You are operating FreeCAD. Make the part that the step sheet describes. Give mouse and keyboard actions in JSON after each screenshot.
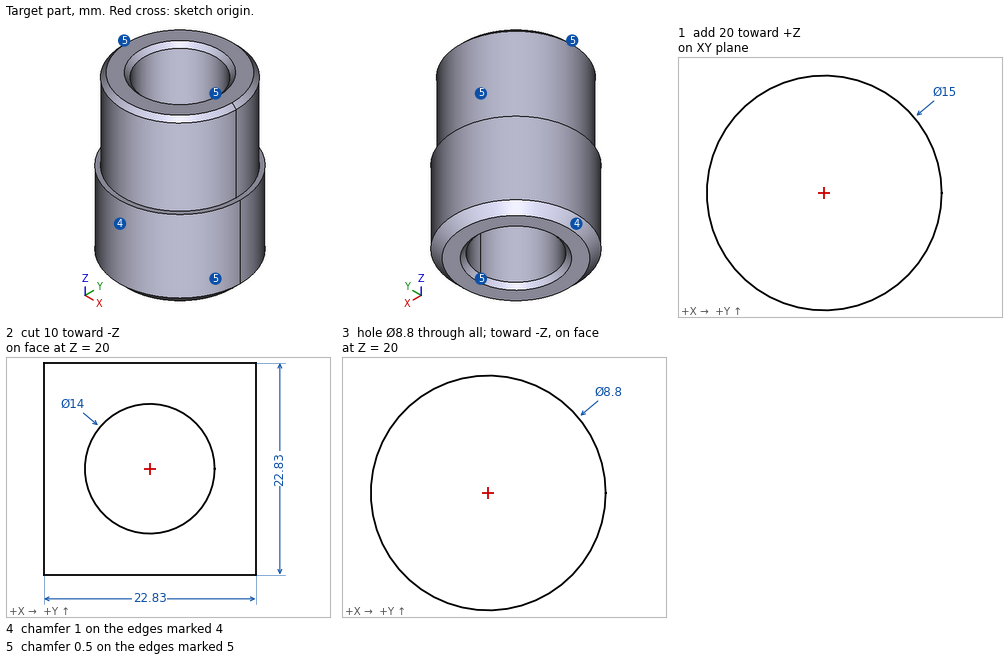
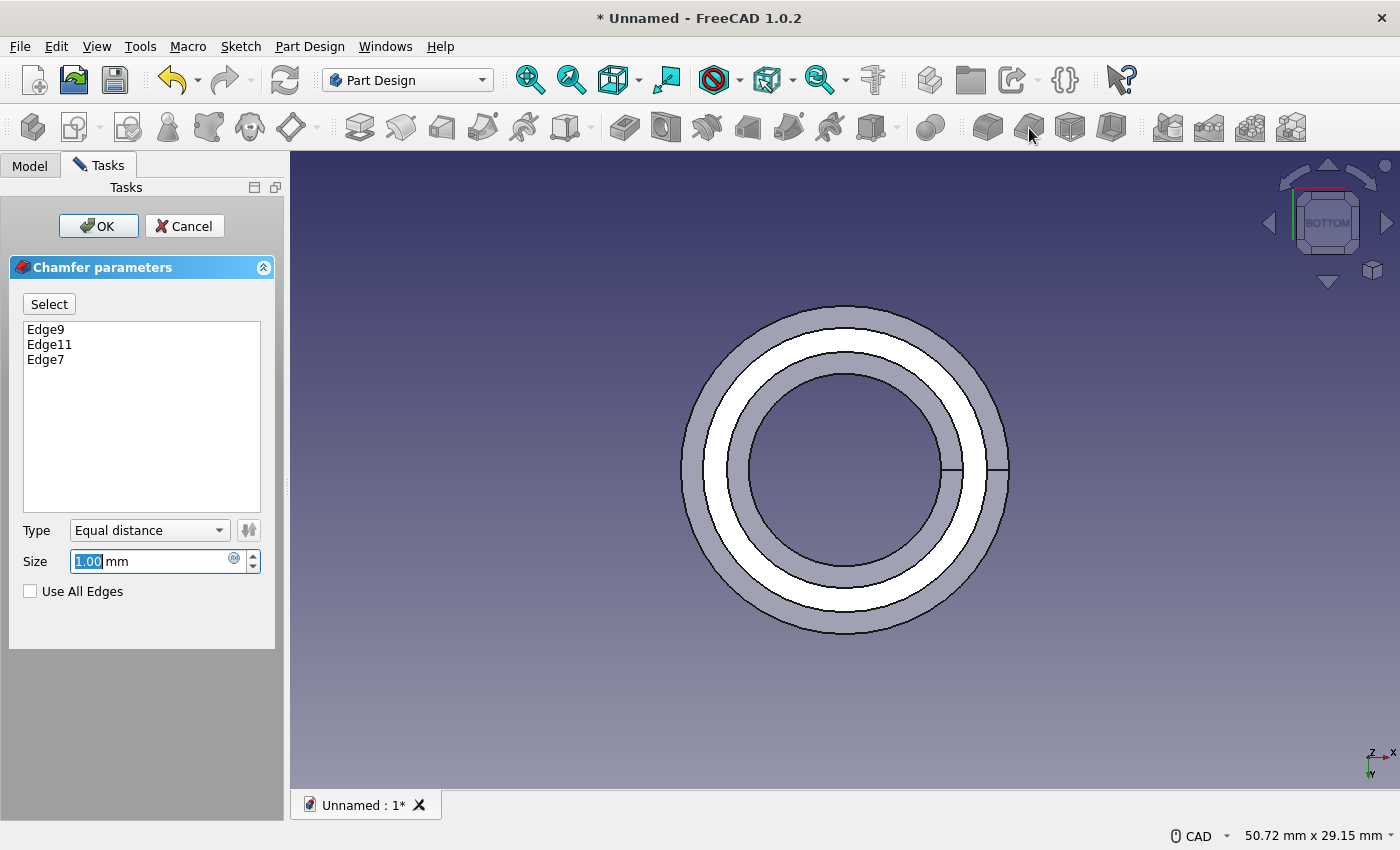
{"action": "type", "text": "0.5"}
{"action": "key", "text": "Tab"}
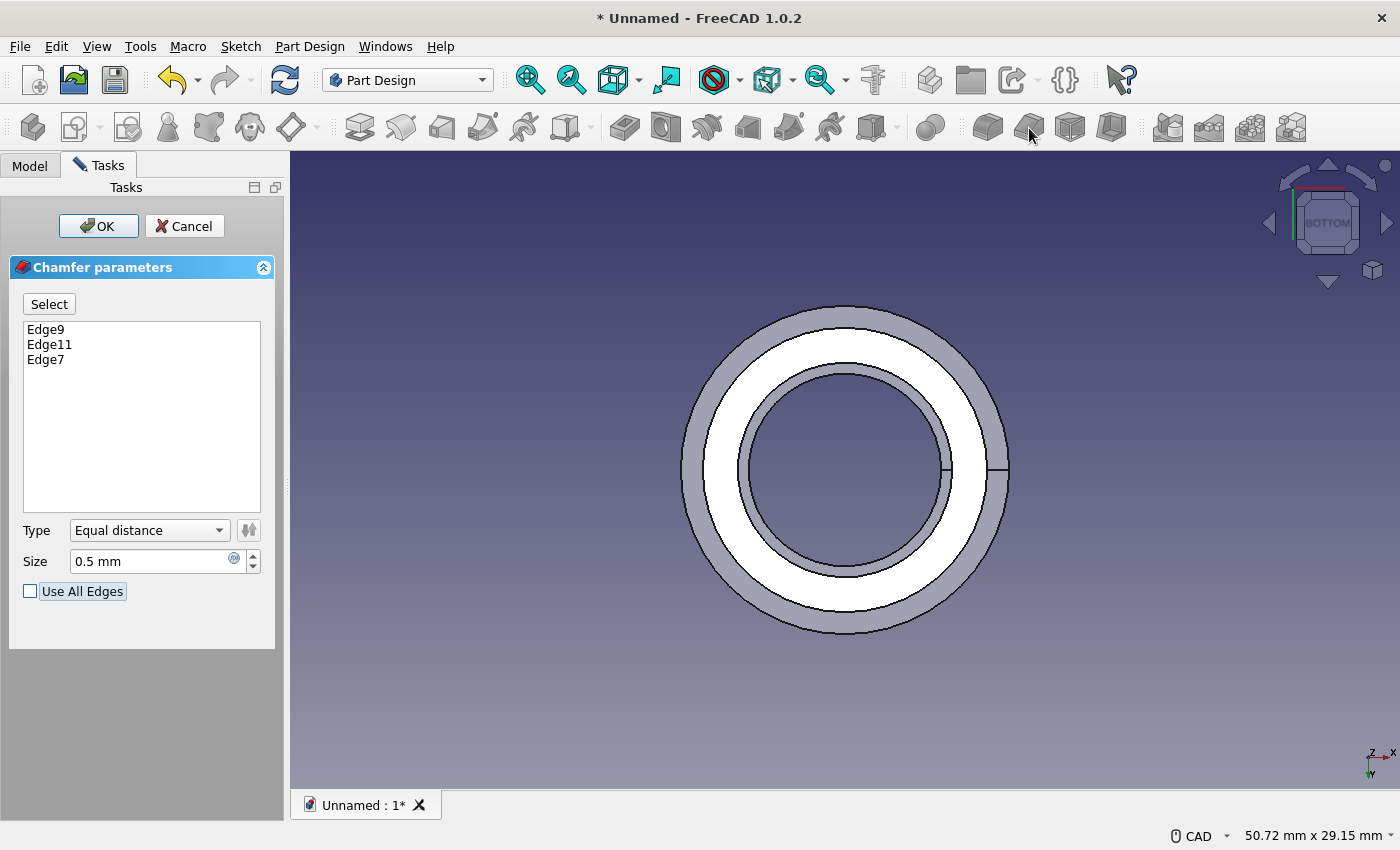
{"action": "left_click", "coordinate": [99, 226]}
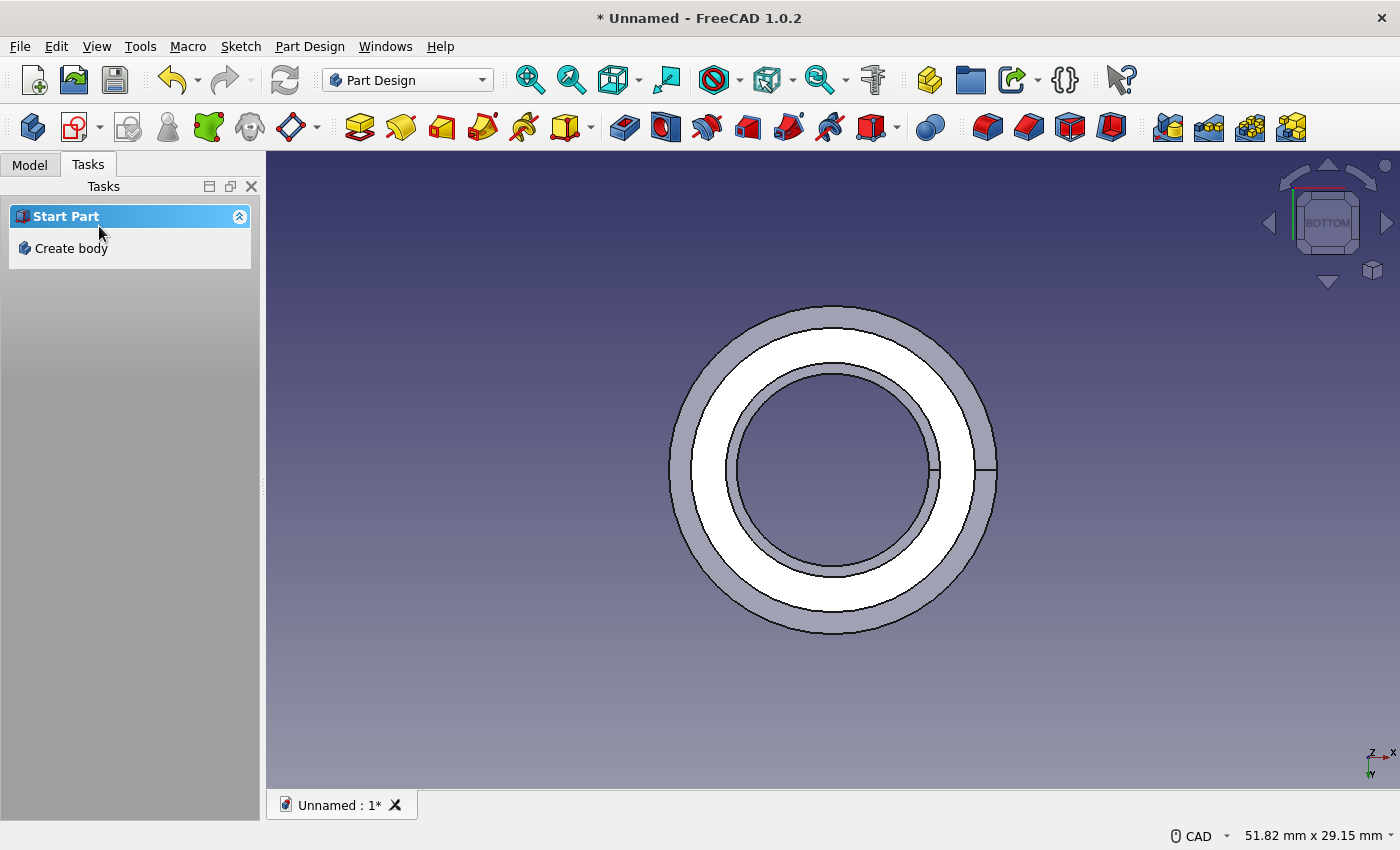
{"action": "key", "text": "0"}